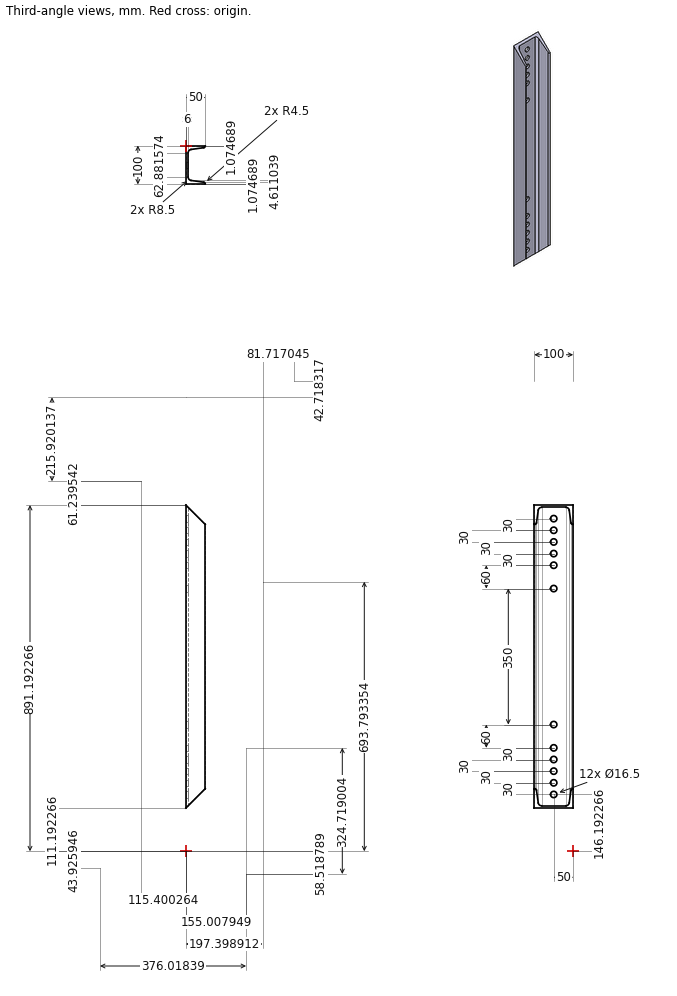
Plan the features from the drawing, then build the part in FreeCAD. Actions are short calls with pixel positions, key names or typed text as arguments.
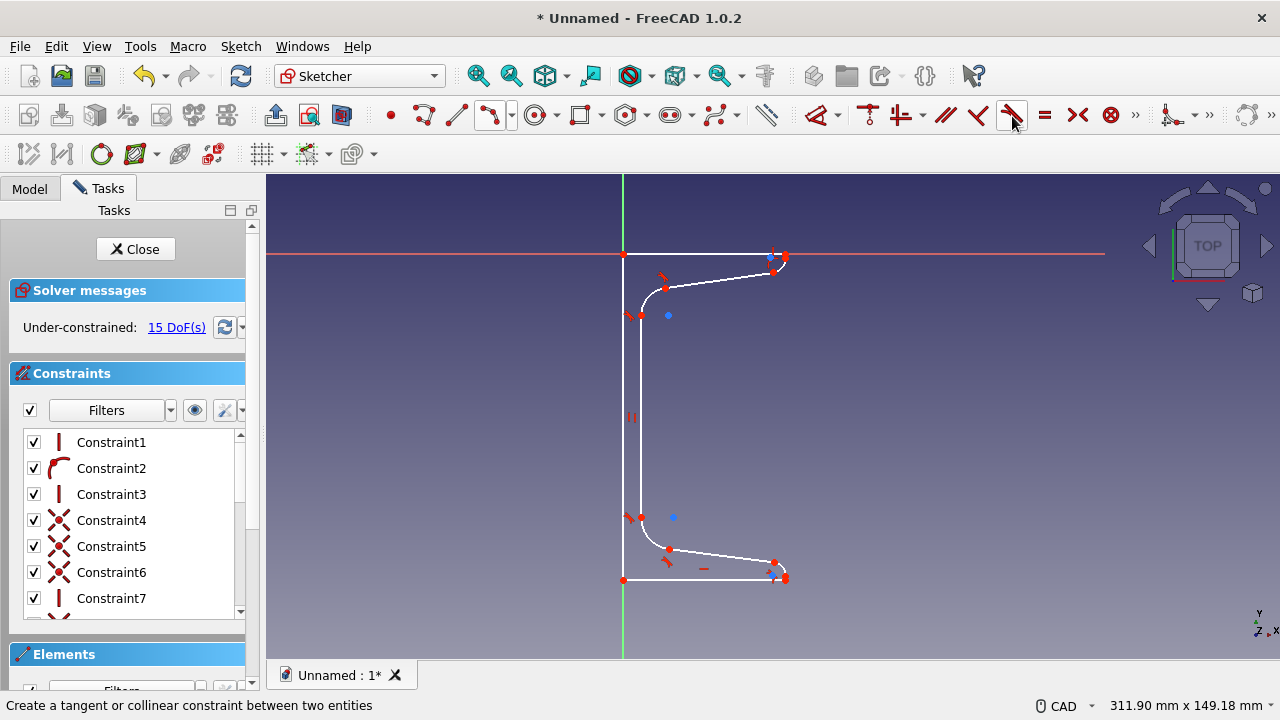
click(698, 284)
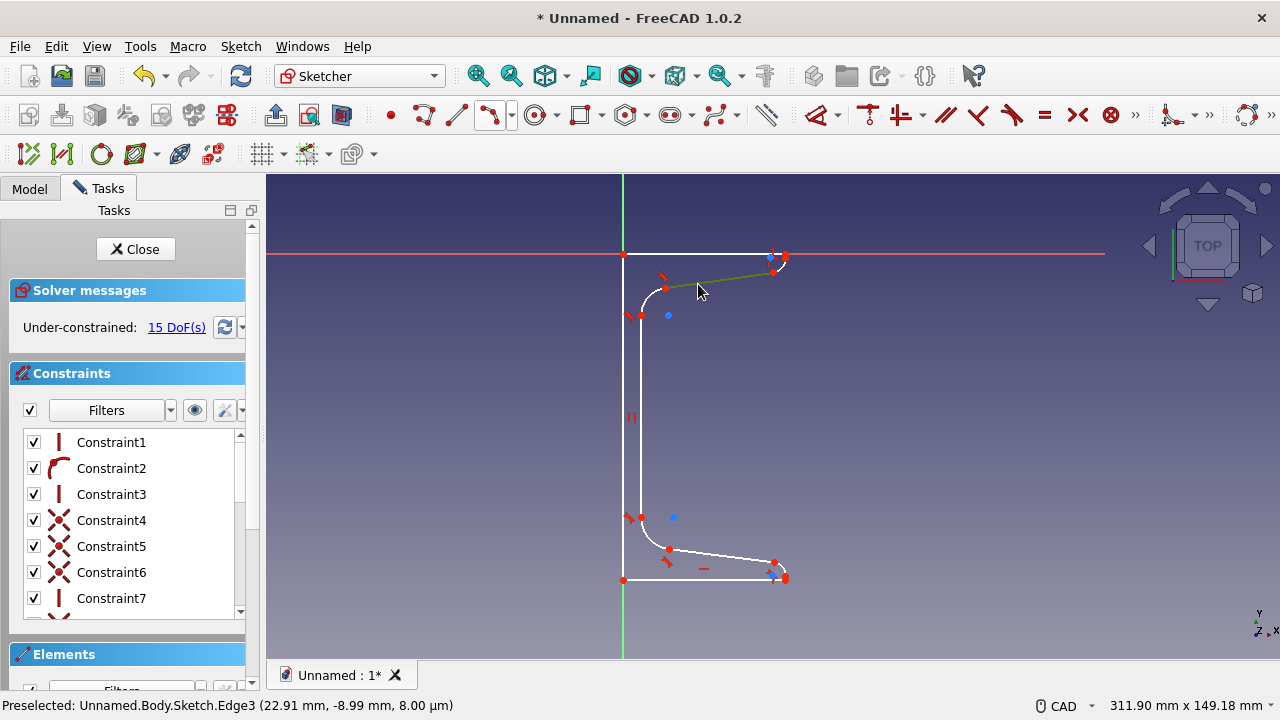
scroll(782, 268, up, 2)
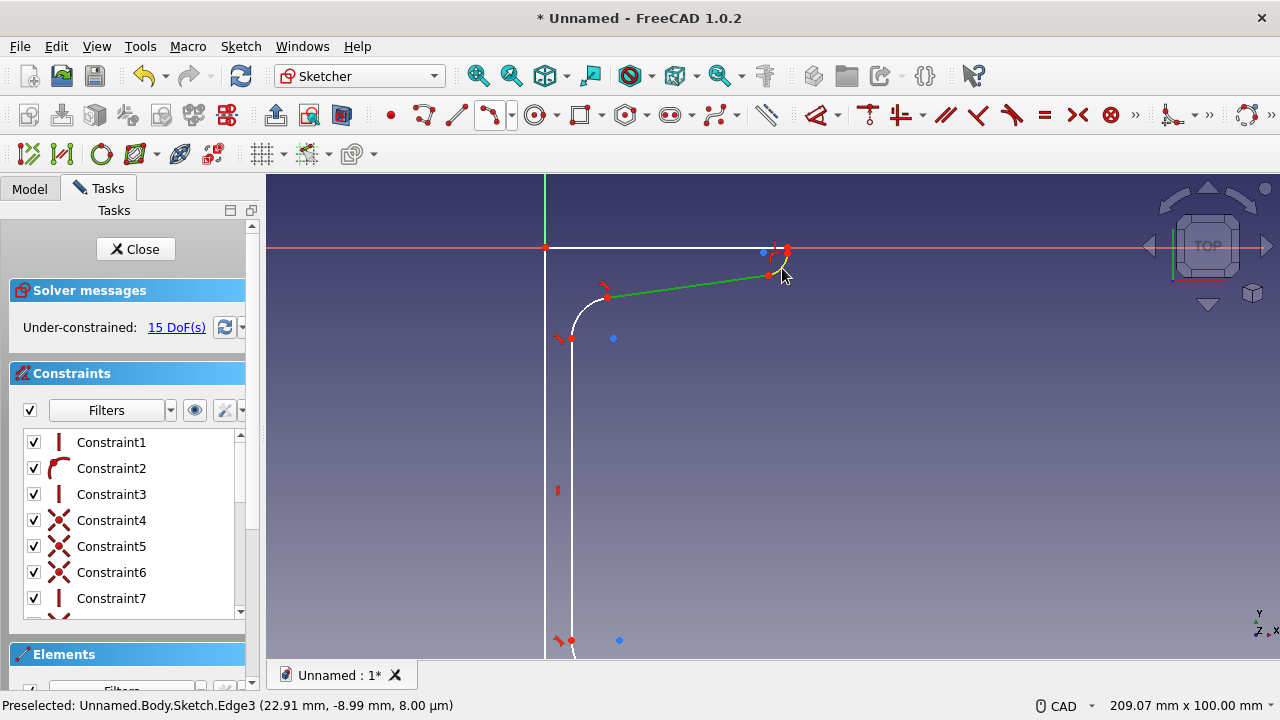
click(782, 267)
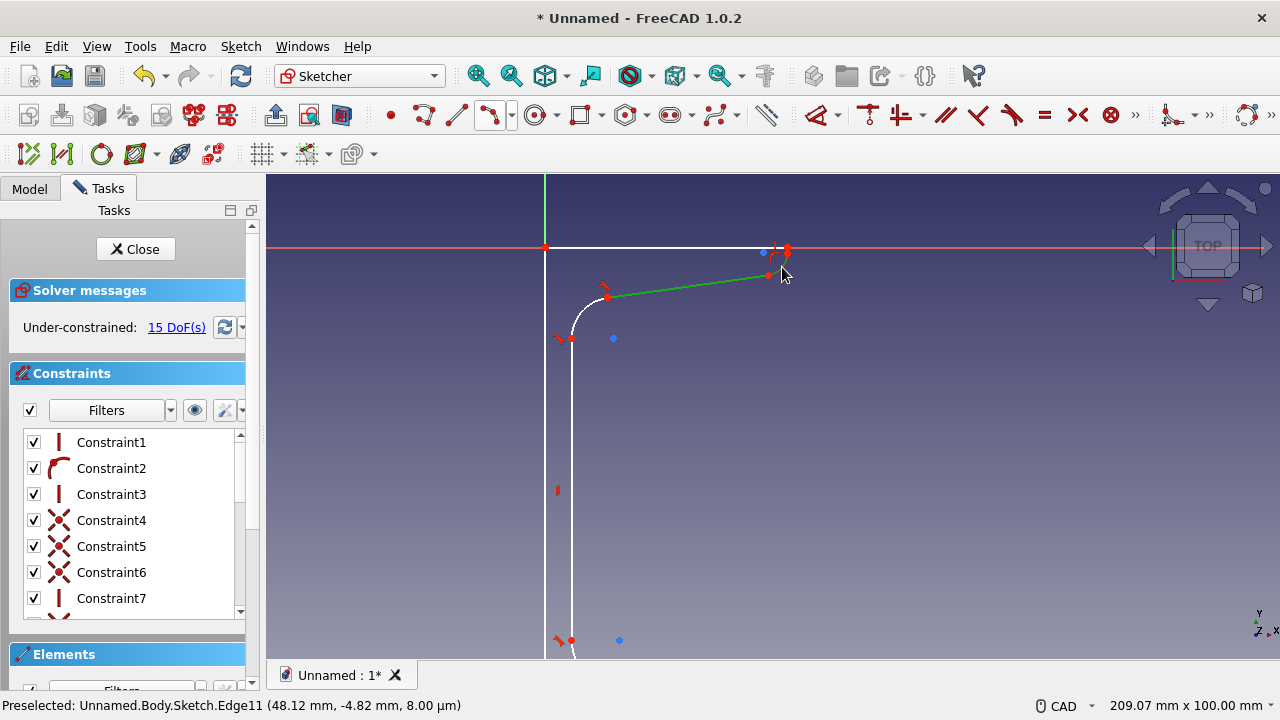
click(1012, 116)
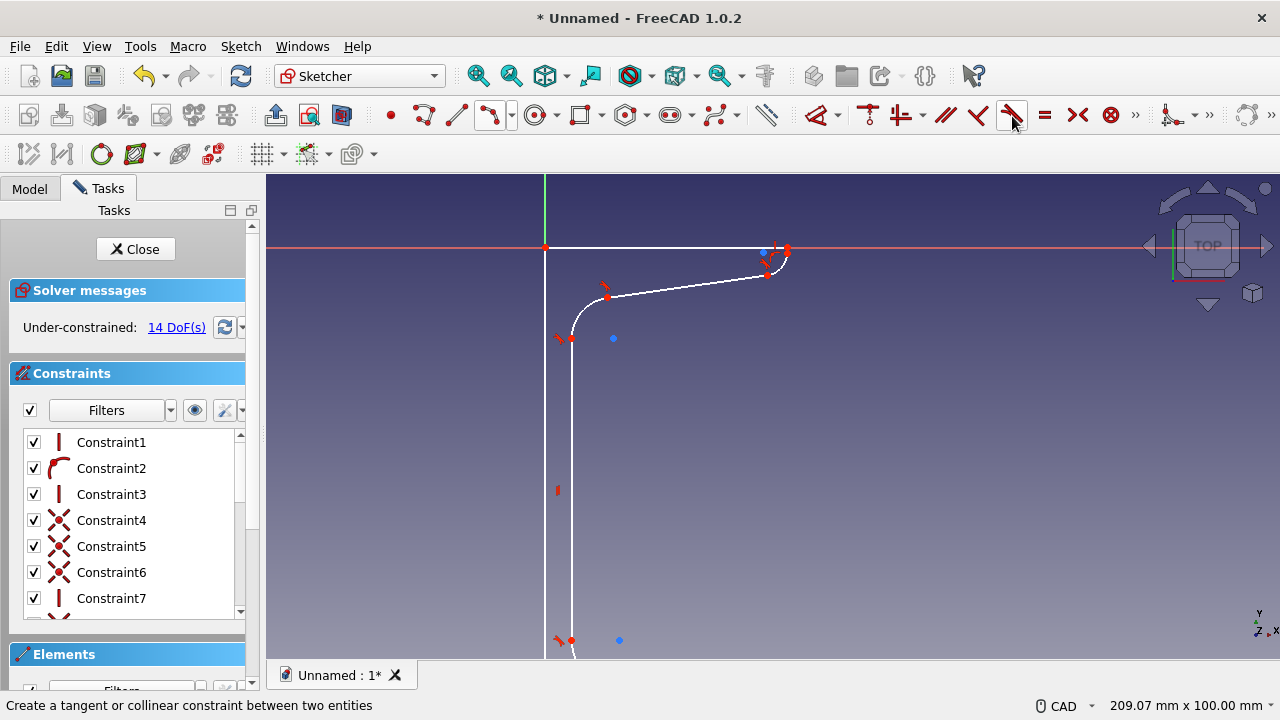
scroll(787, 250, up, 9)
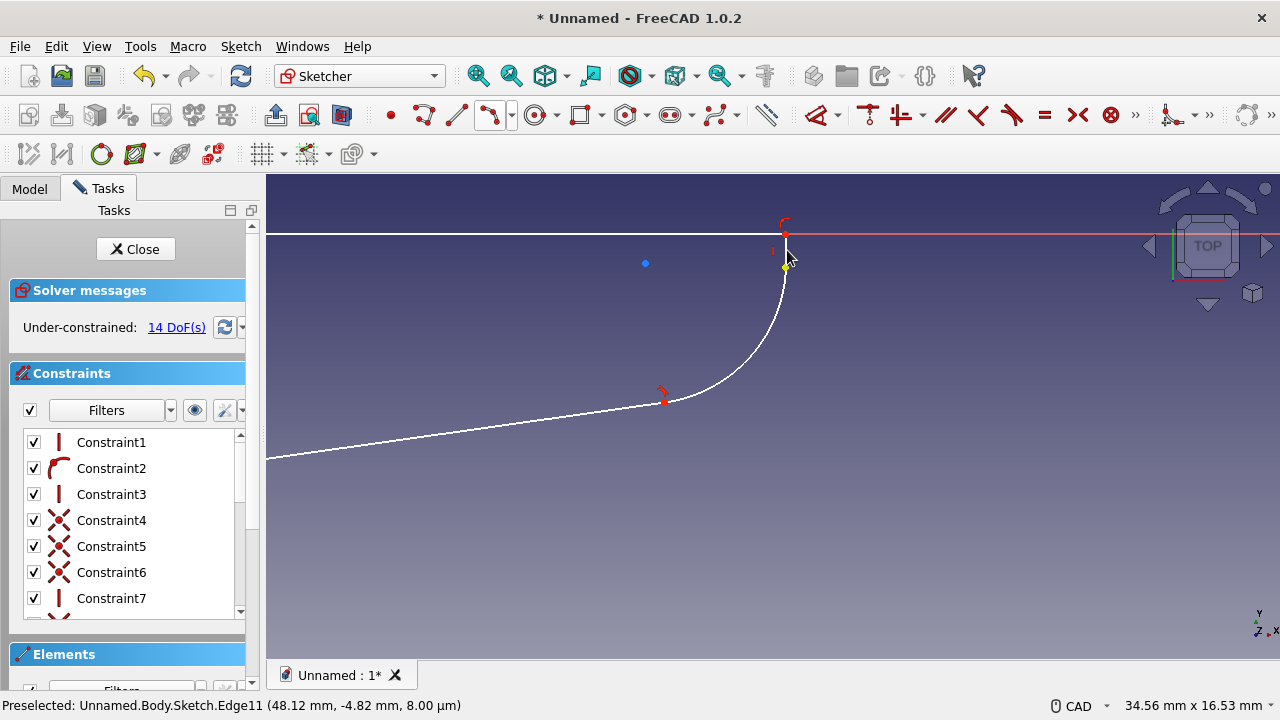
click(786, 251)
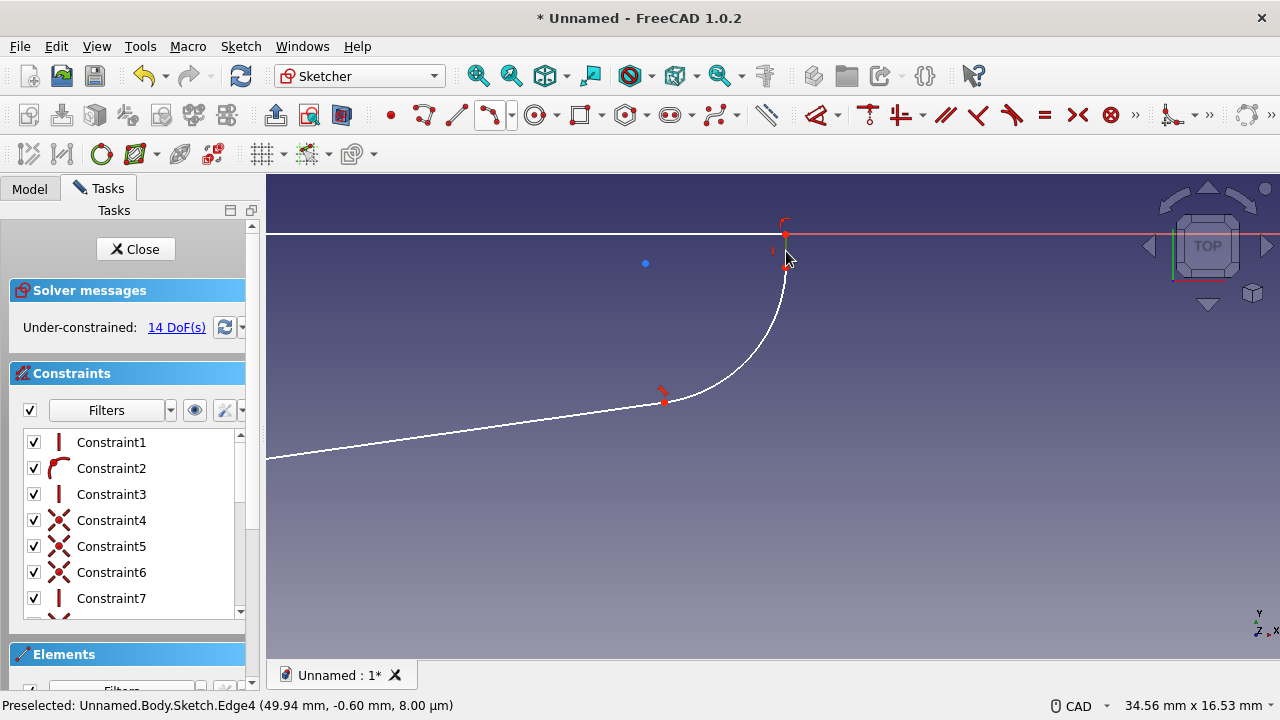
scroll(786, 256, down, 11)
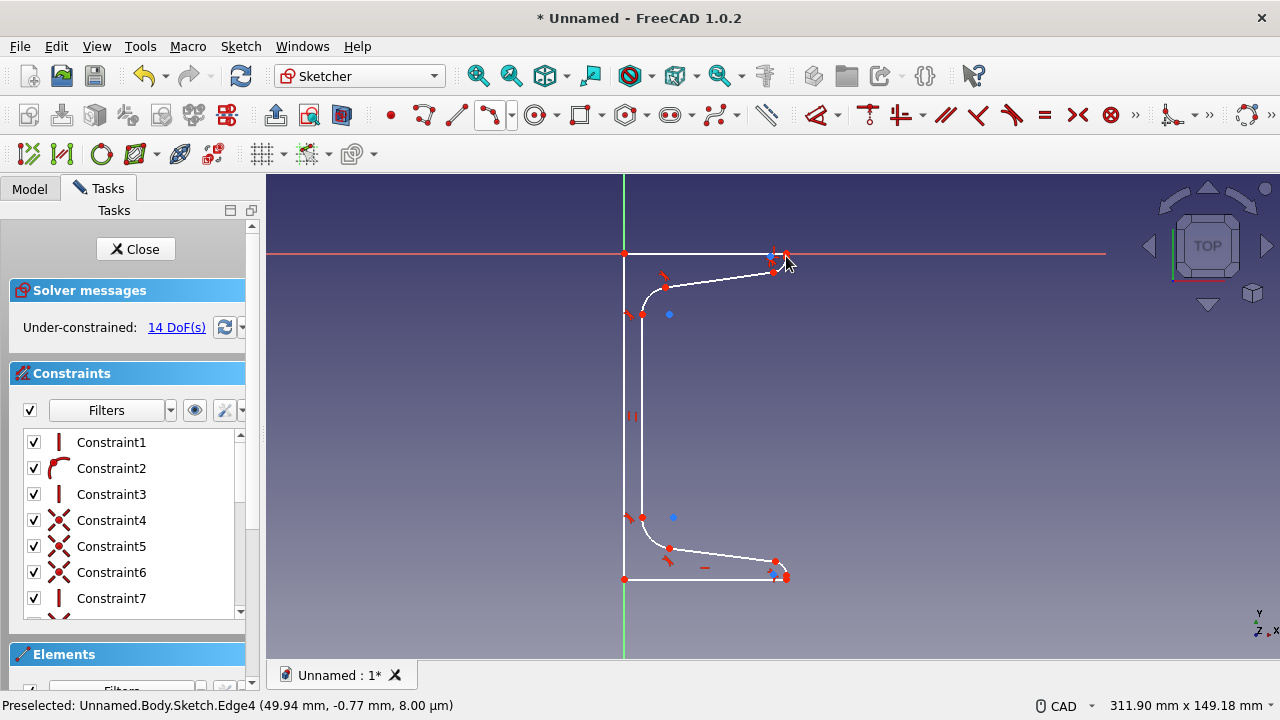
scroll(779, 270, up, 4)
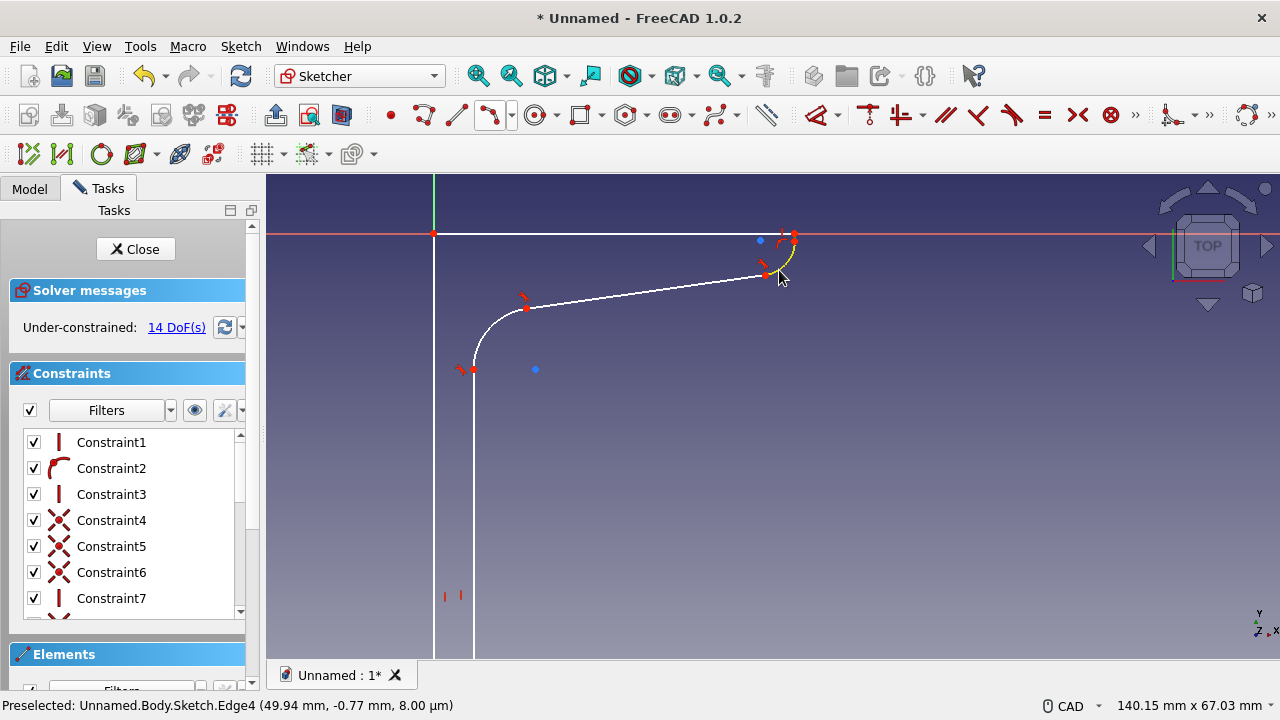
click(779, 270)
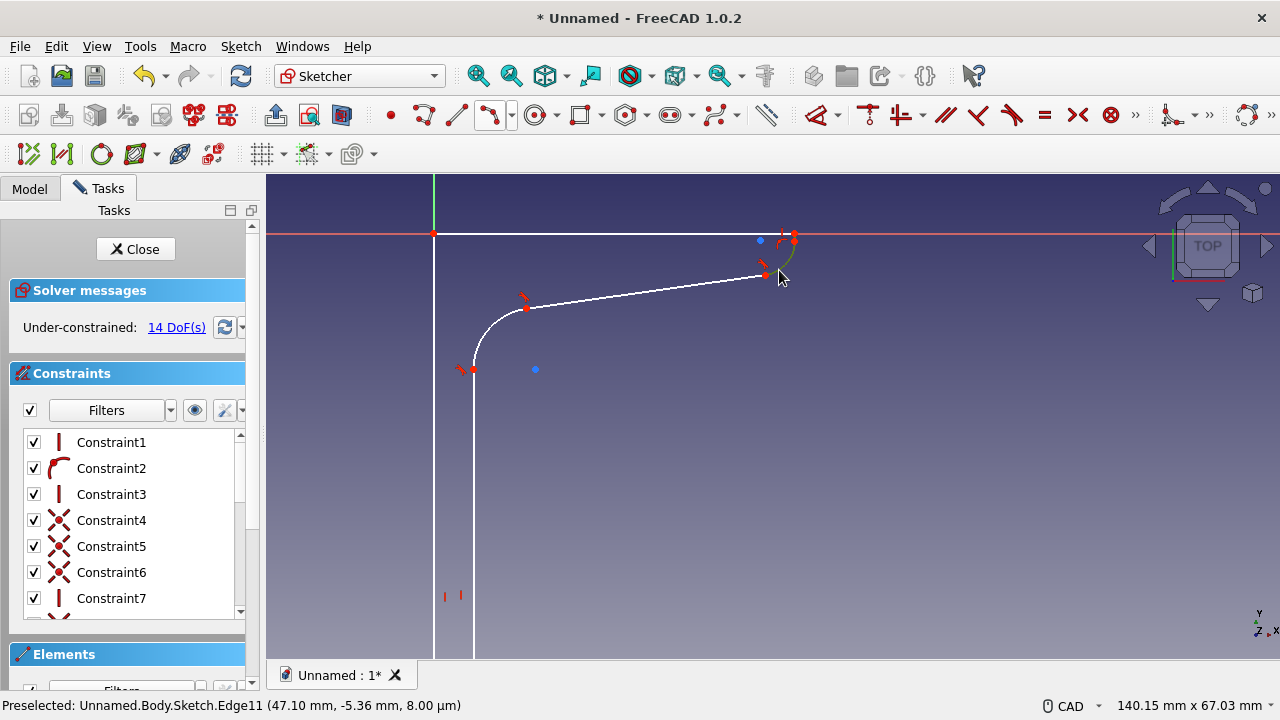
click(1012, 116)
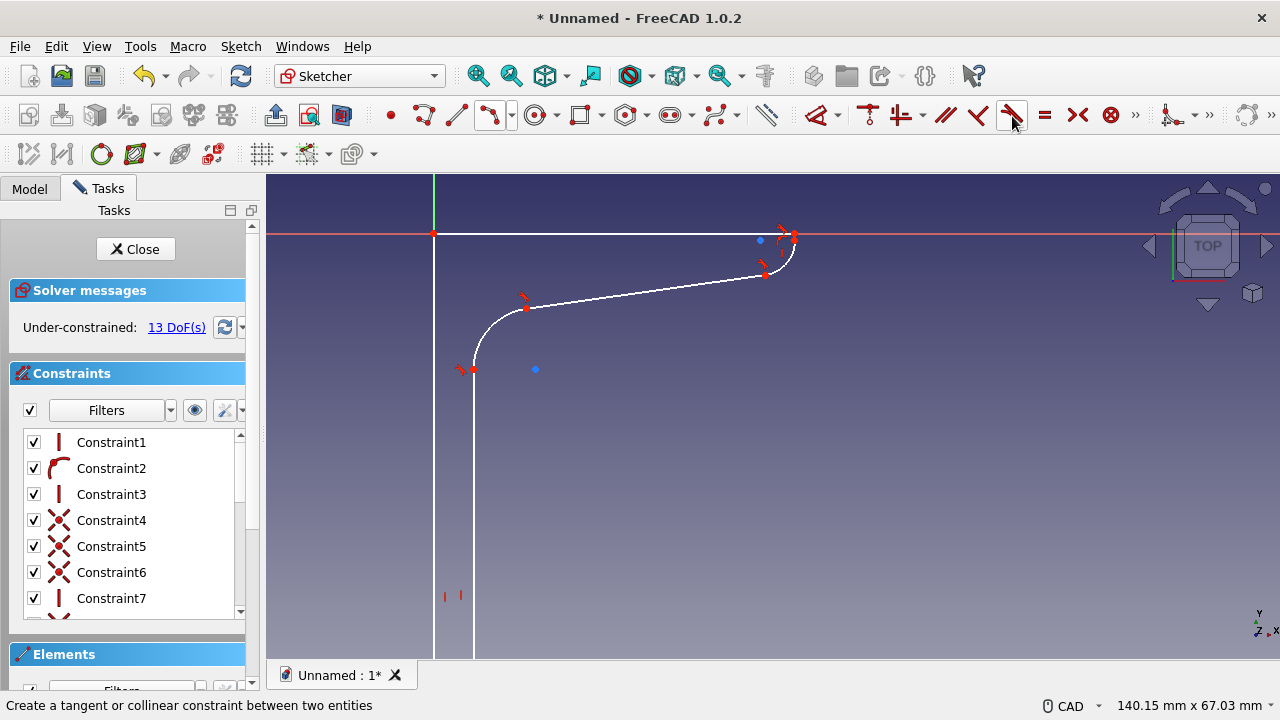
scroll(778, 271, down, 4)